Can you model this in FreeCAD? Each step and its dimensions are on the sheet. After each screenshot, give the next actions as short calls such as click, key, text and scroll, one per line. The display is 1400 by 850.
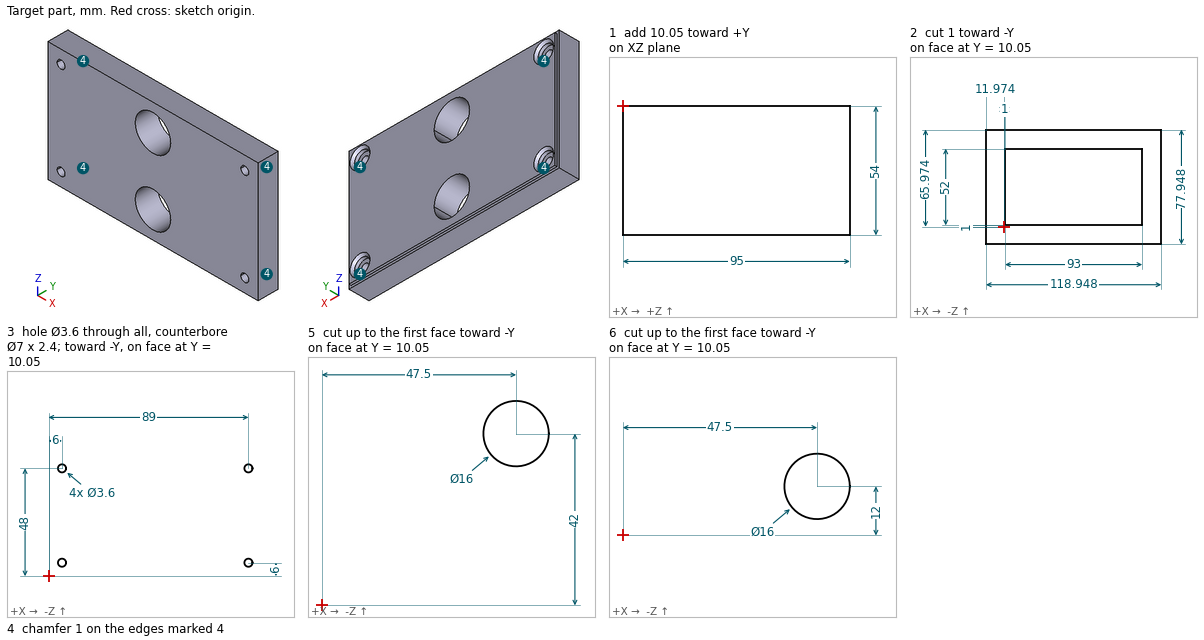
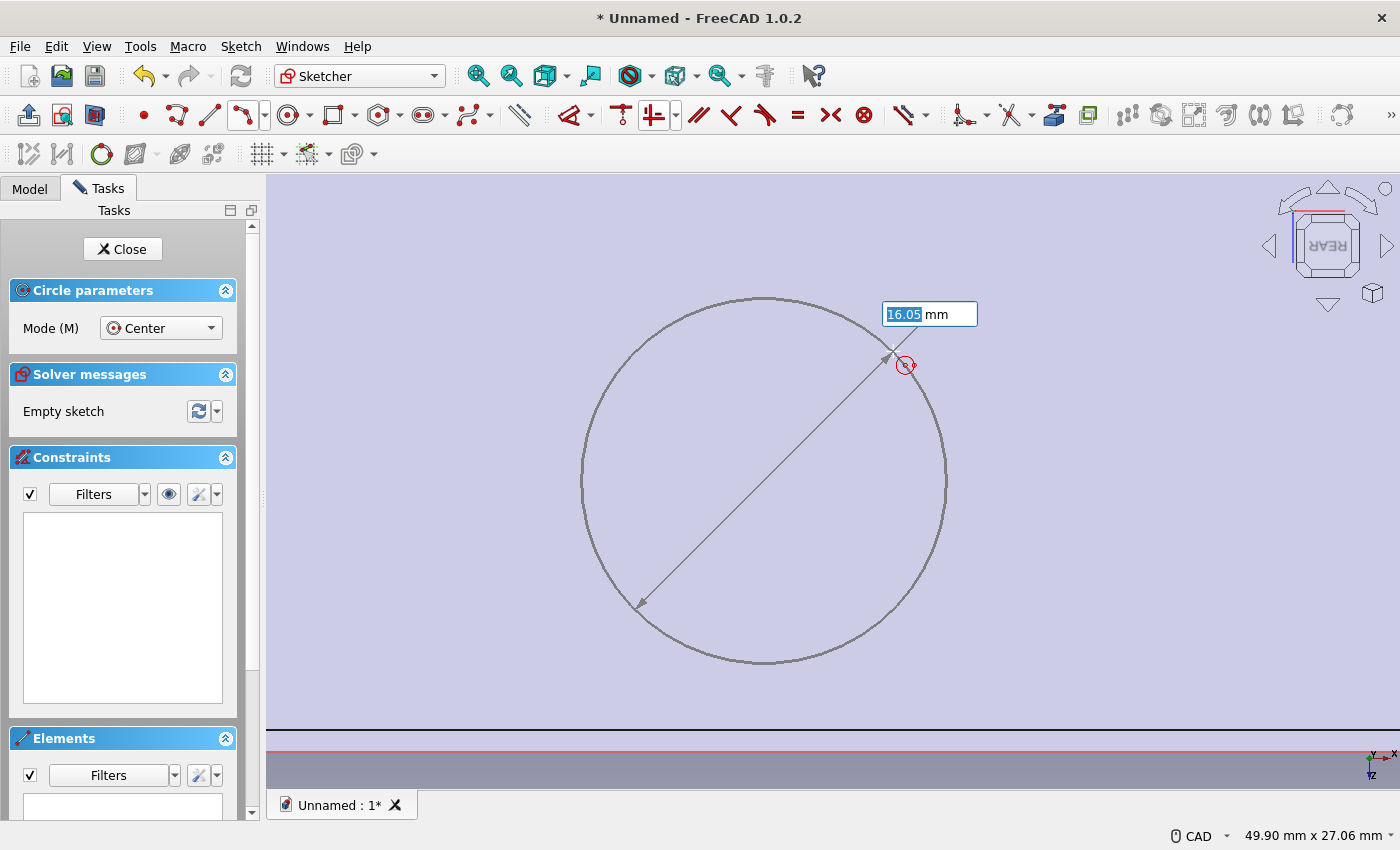
text(16)
key(Return)
key(Escape)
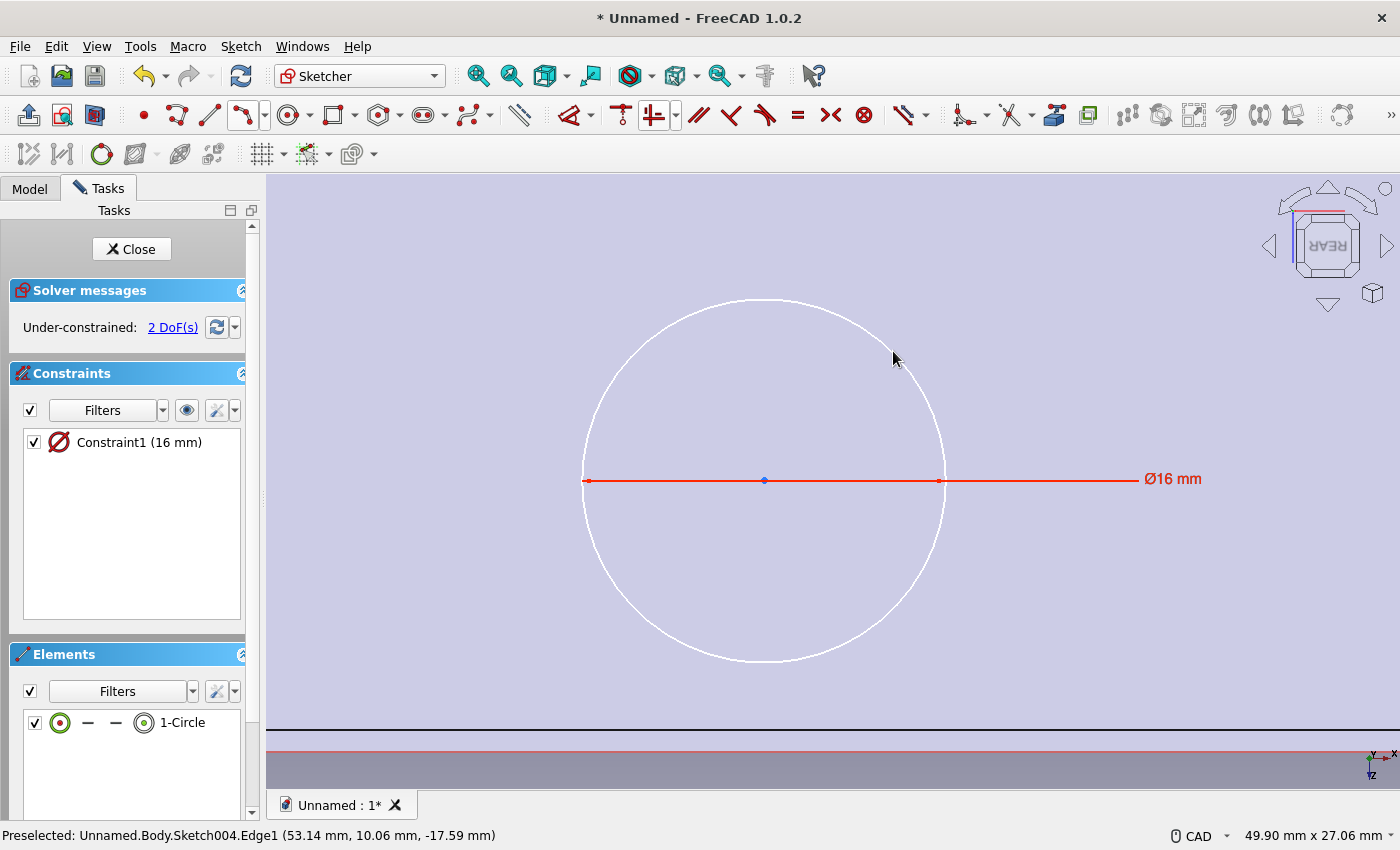
click(568, 116)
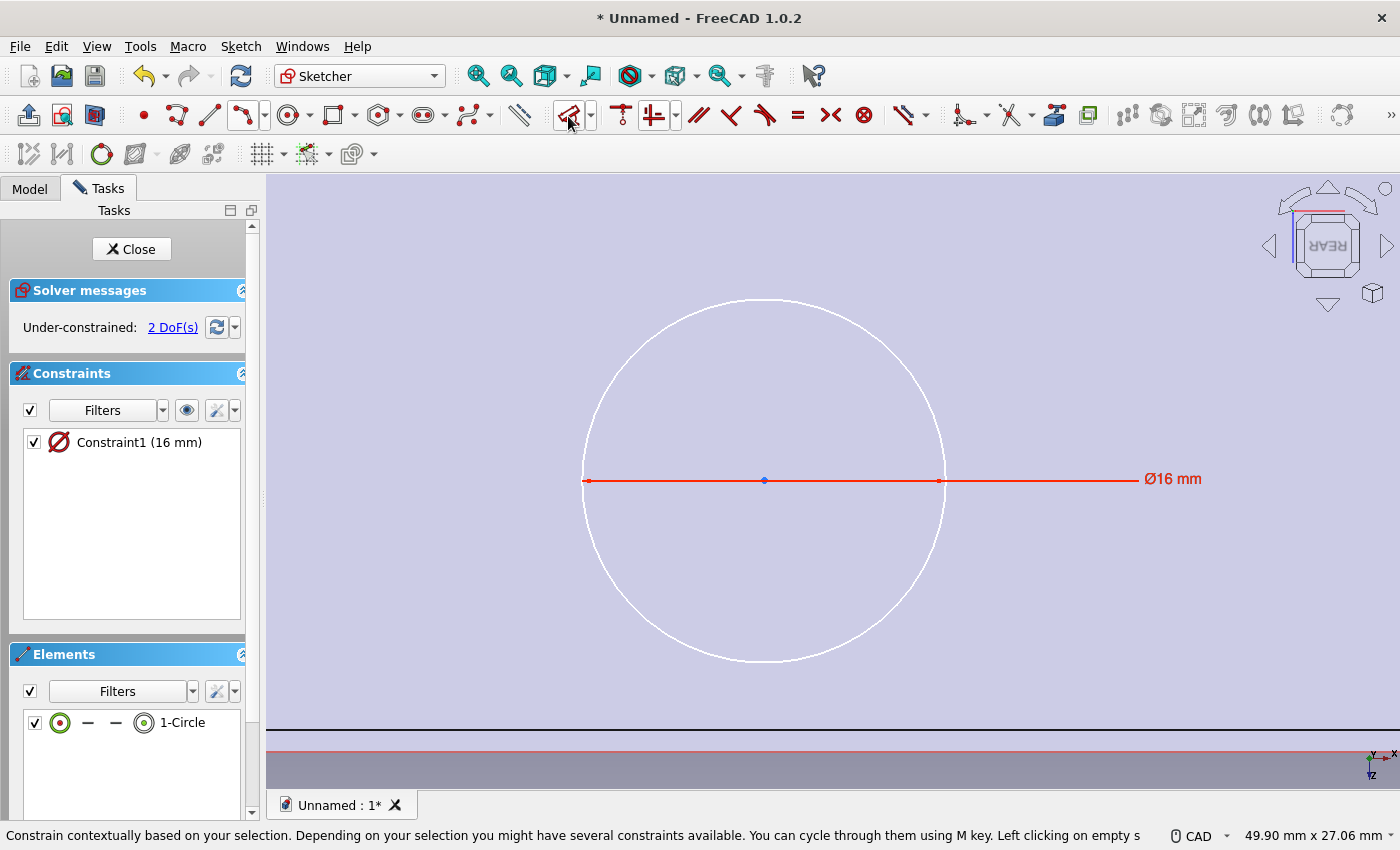
click(764, 481)
click(798, 617)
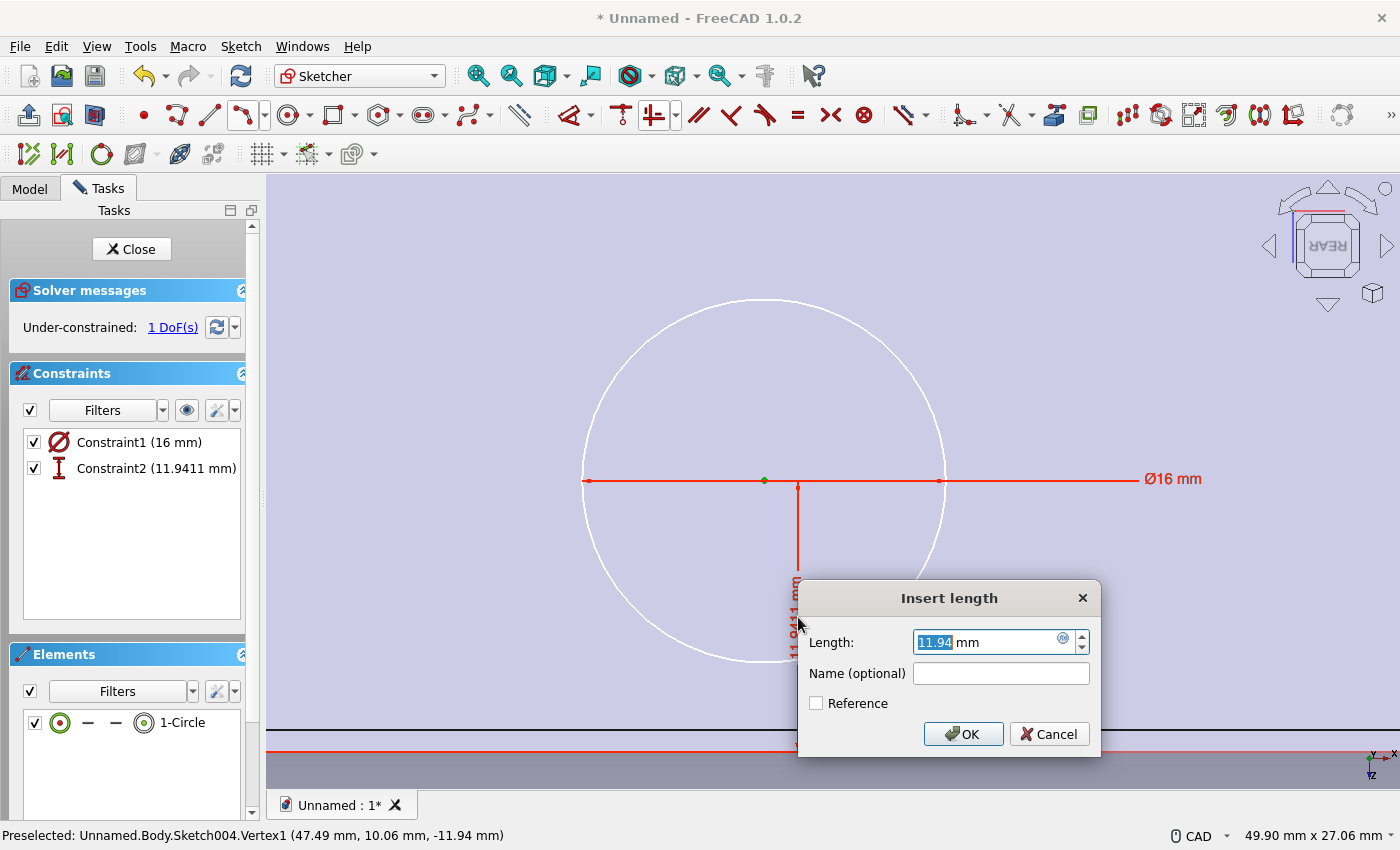
text(12)
key(Return)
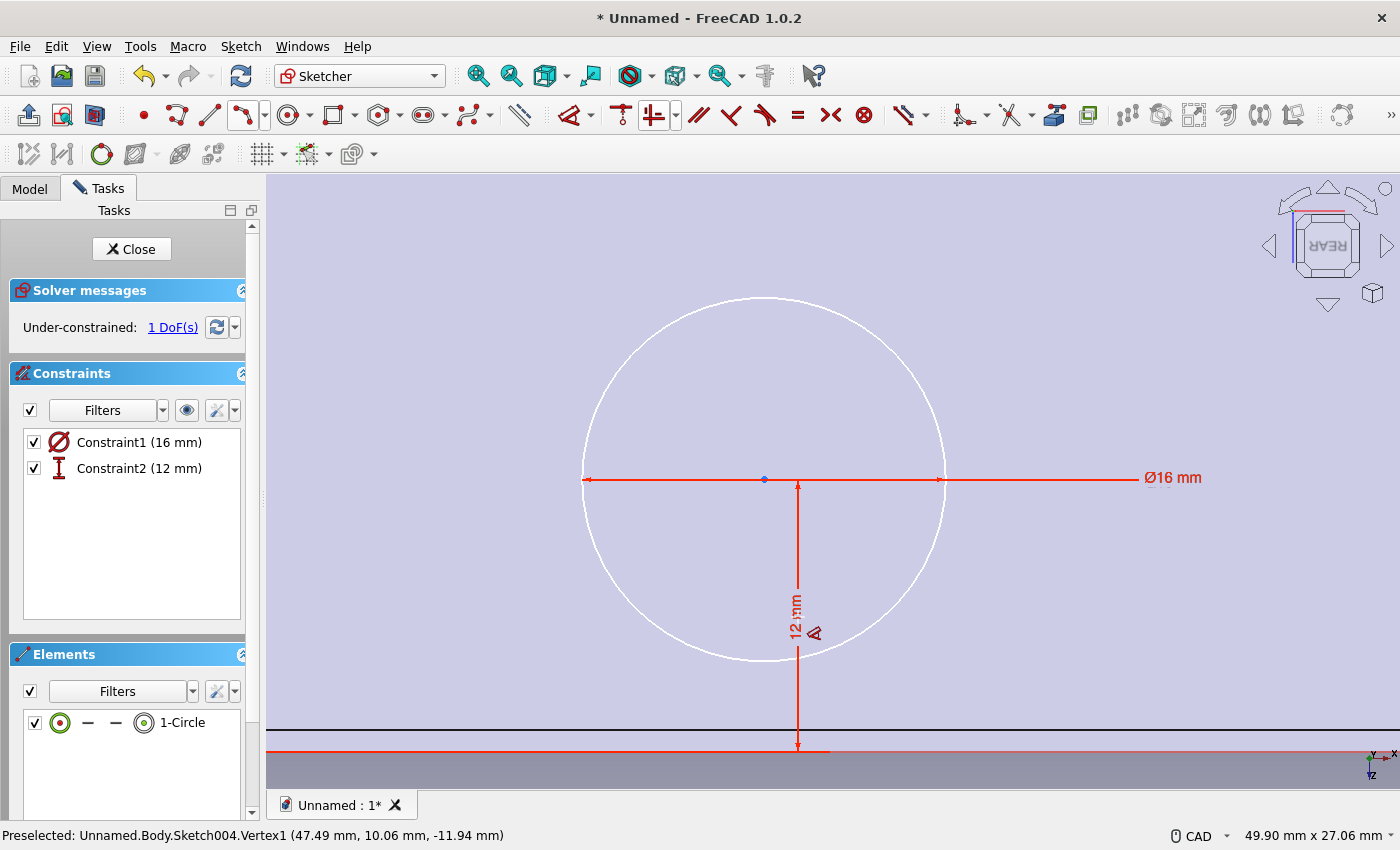
click(764, 480)
click(529, 446)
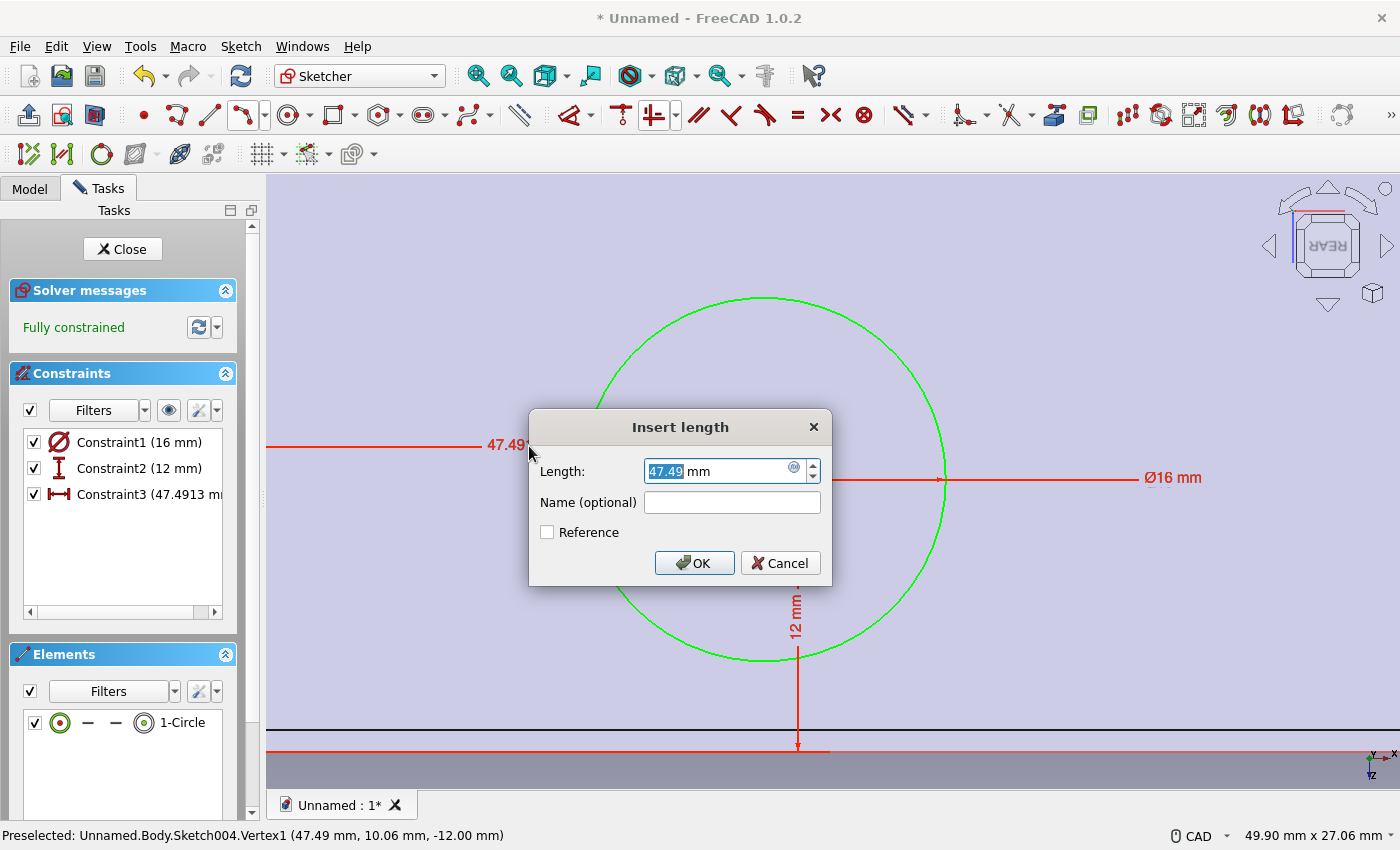
text(47.5)
key(Return)
key(Escape)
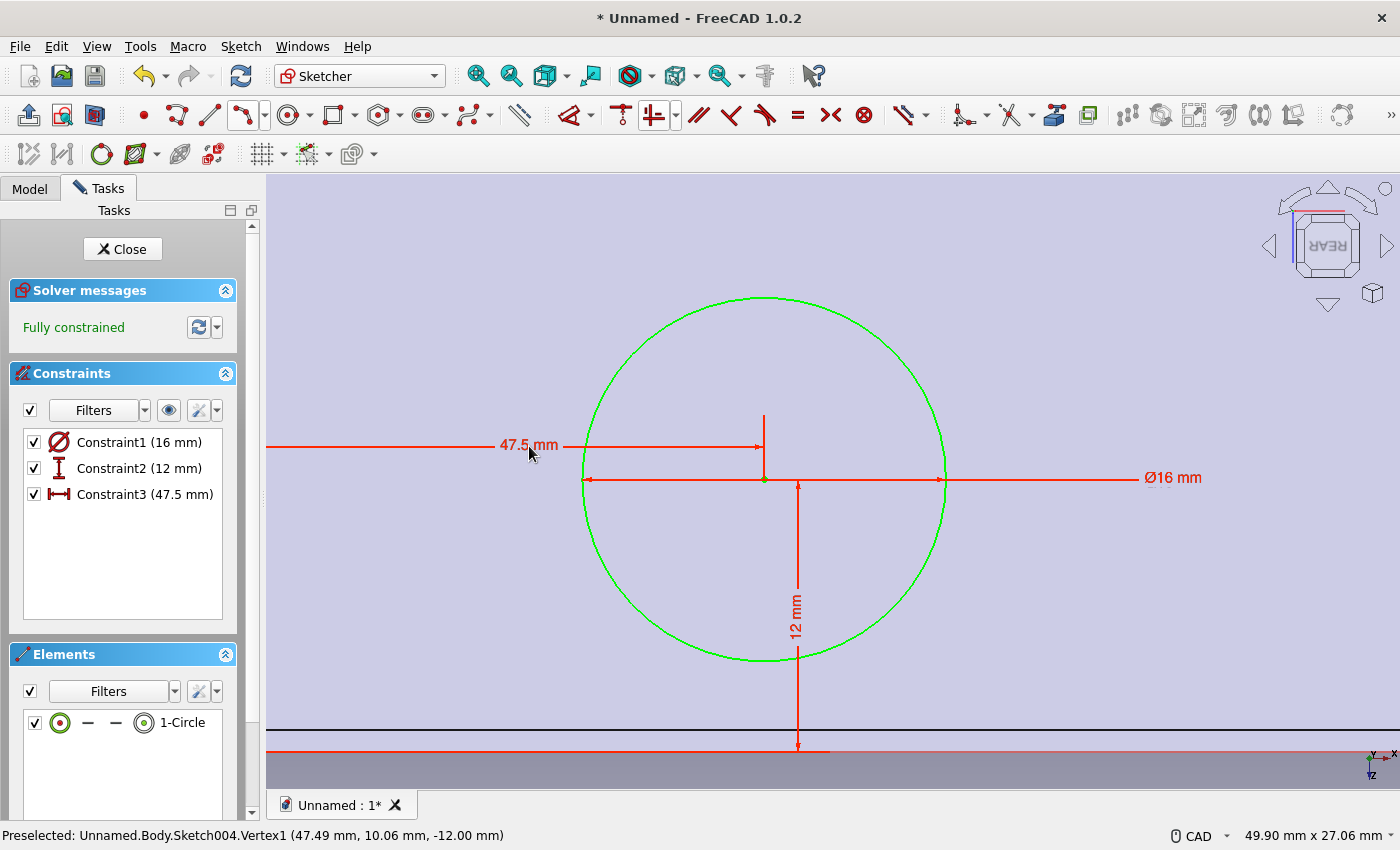
click(123, 249)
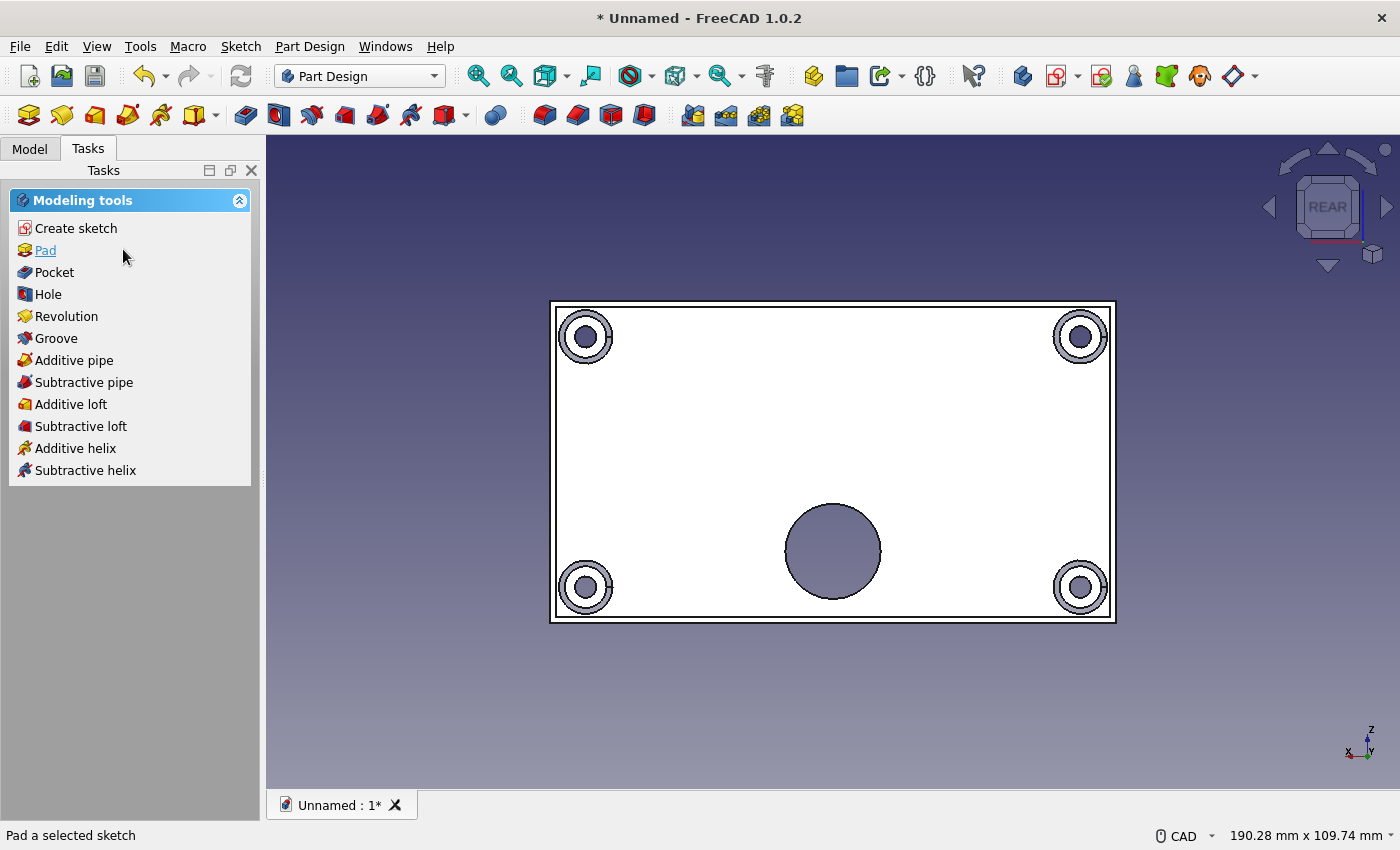
click(246, 116)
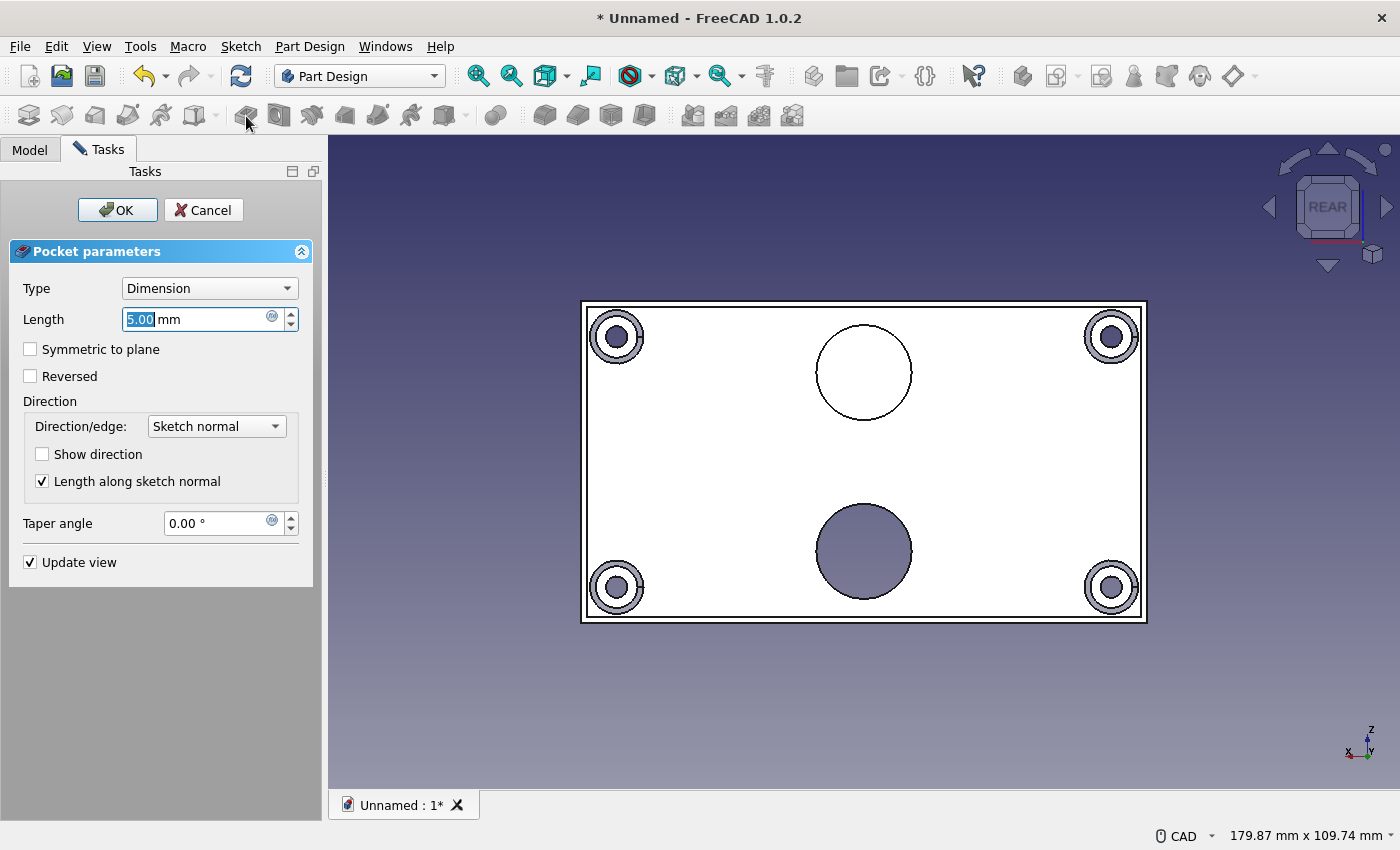
click(210, 288)